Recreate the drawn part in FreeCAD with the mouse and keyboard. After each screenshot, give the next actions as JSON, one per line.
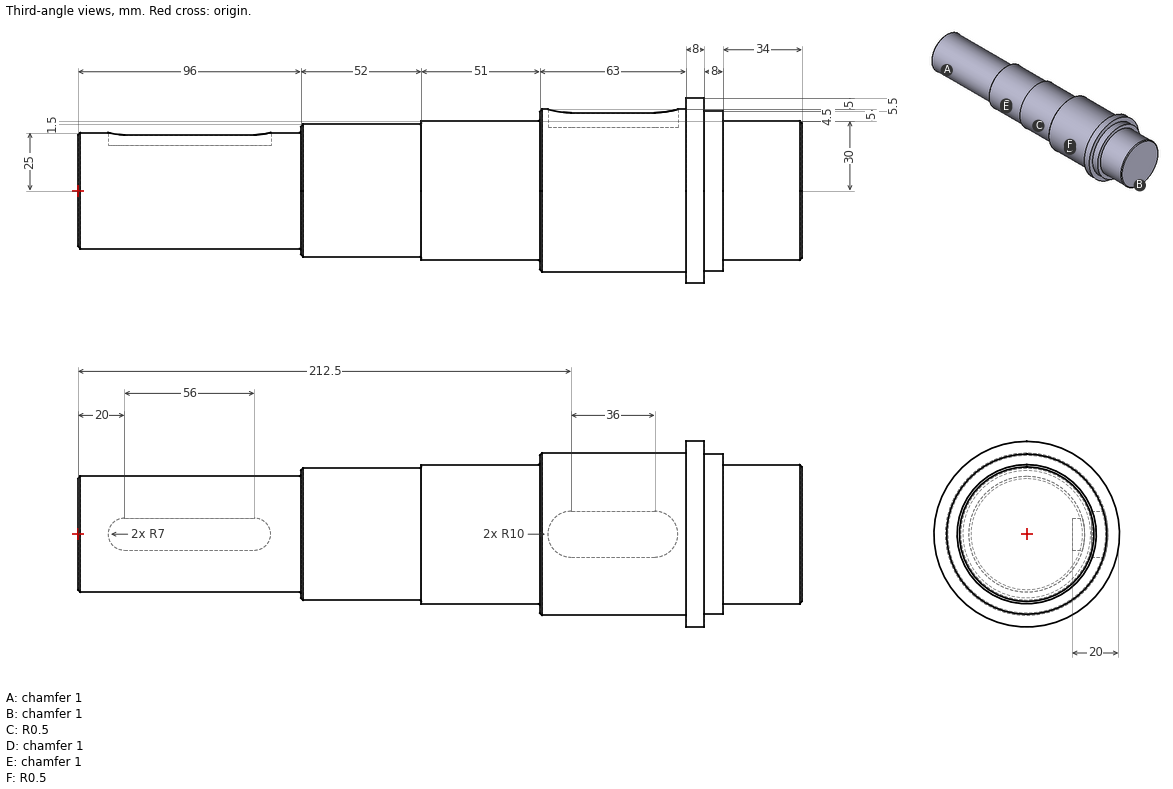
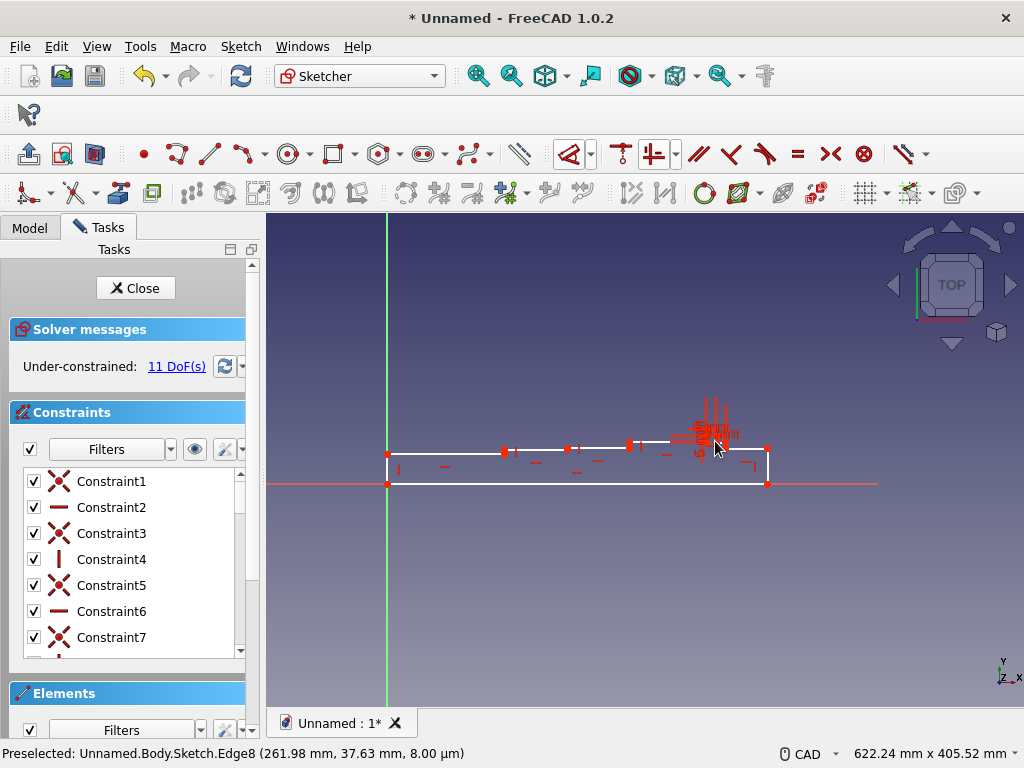
{"action": "scroll", "coordinate": [630, 444], "scroll_direction": "up", "scroll_amount": 11}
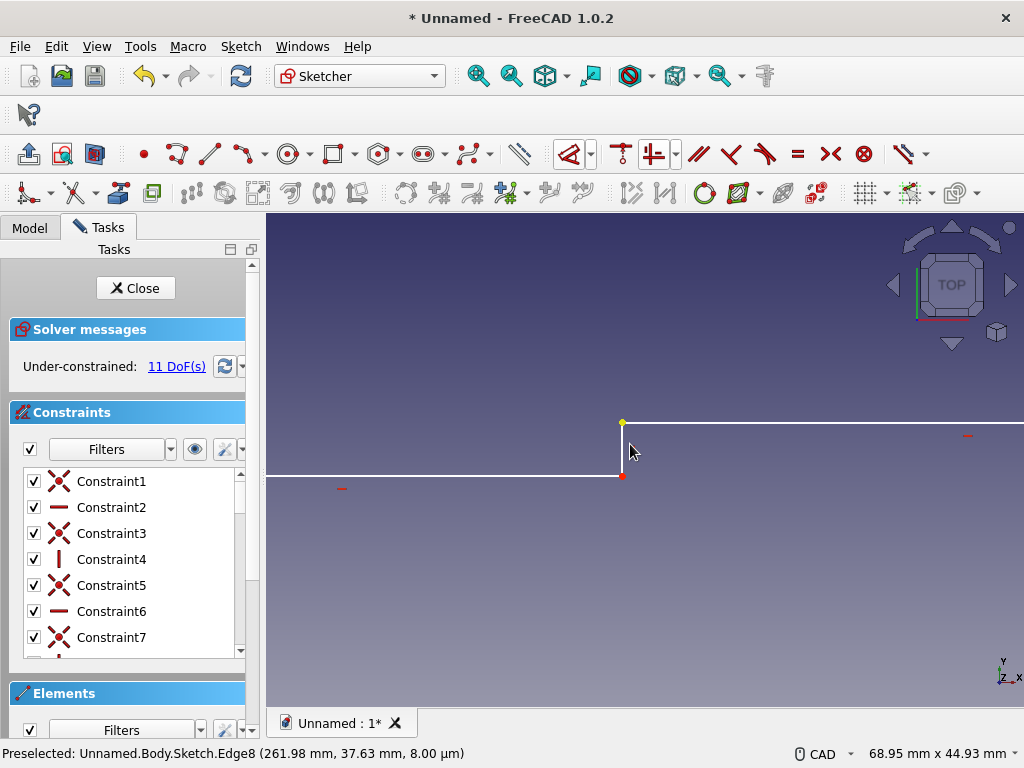
{"action": "left_click", "coordinate": [622, 439]}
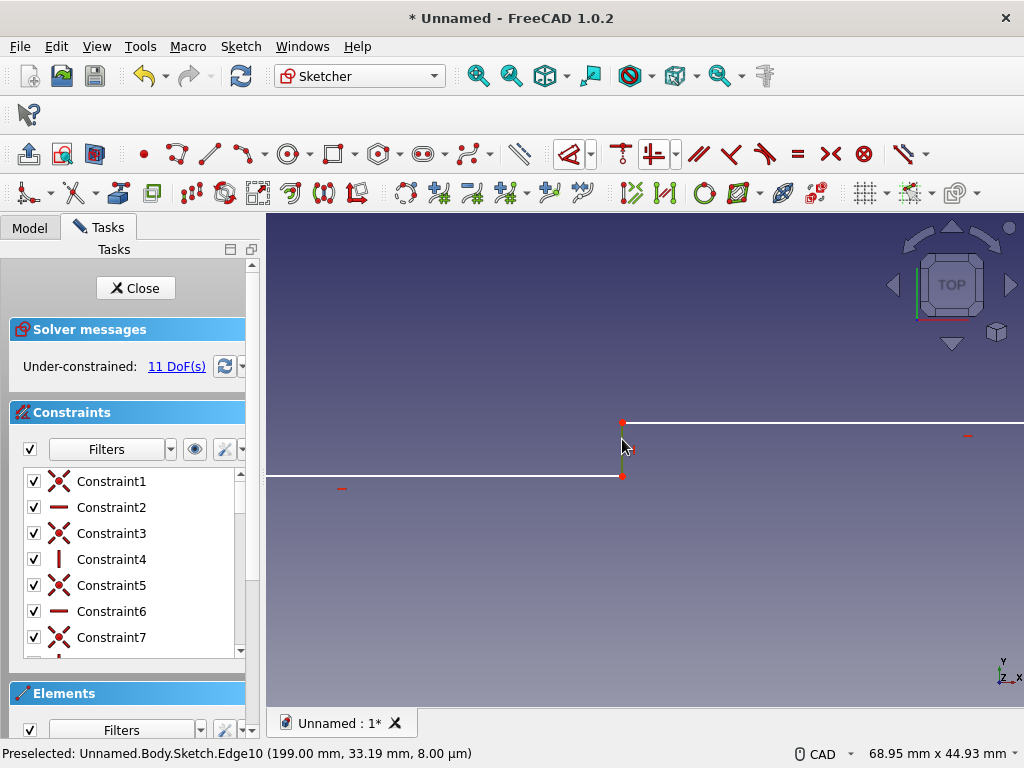
{"action": "key", "text": "i"}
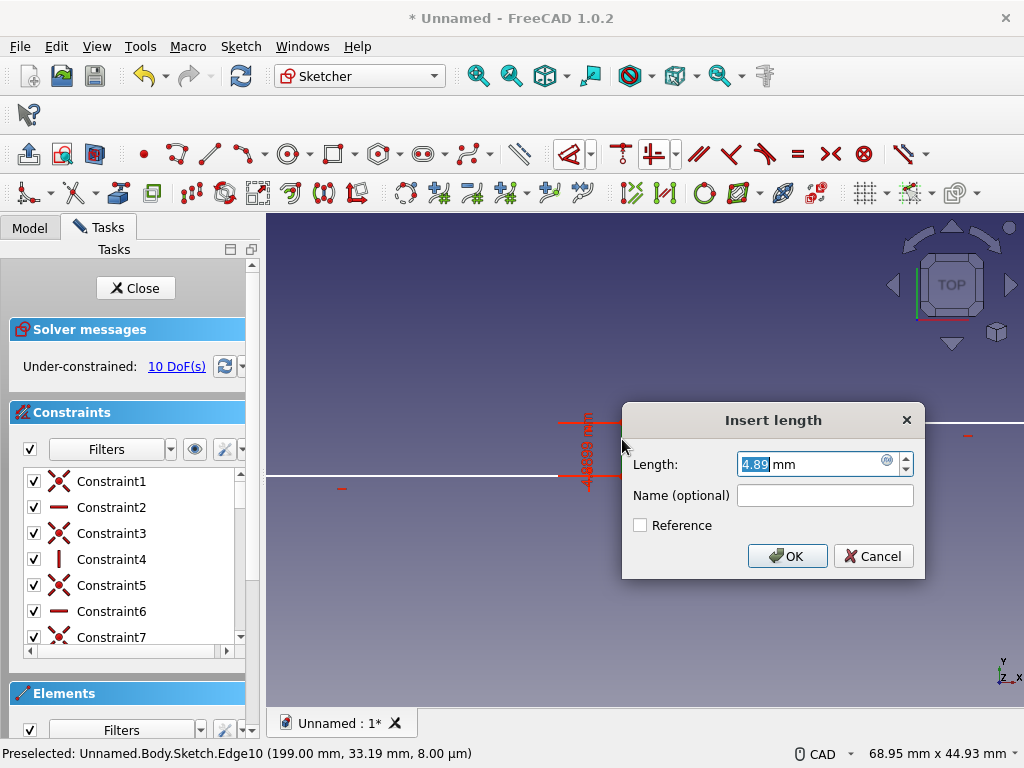
{"action": "type", "text": "5"}
{"action": "key", "text": "Return"}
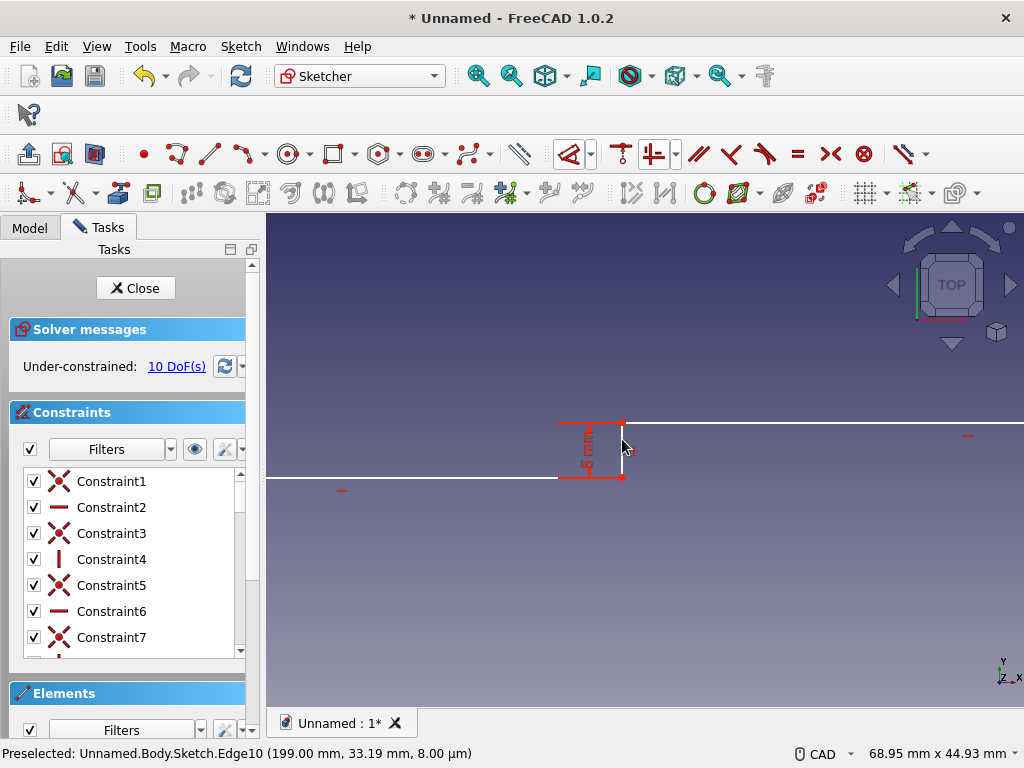
{"action": "scroll", "coordinate": [630, 444], "scroll_direction": "down", "scroll_amount": 11}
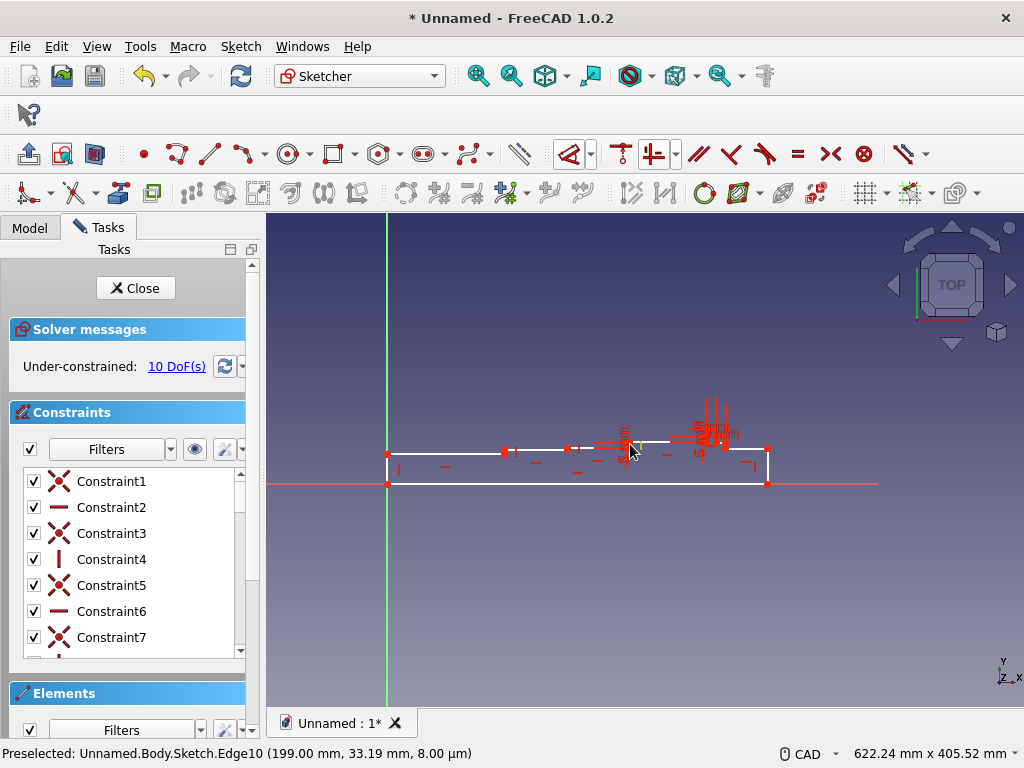
{"action": "scroll", "coordinate": [768, 474], "scroll_direction": "up", "scroll_amount": 2}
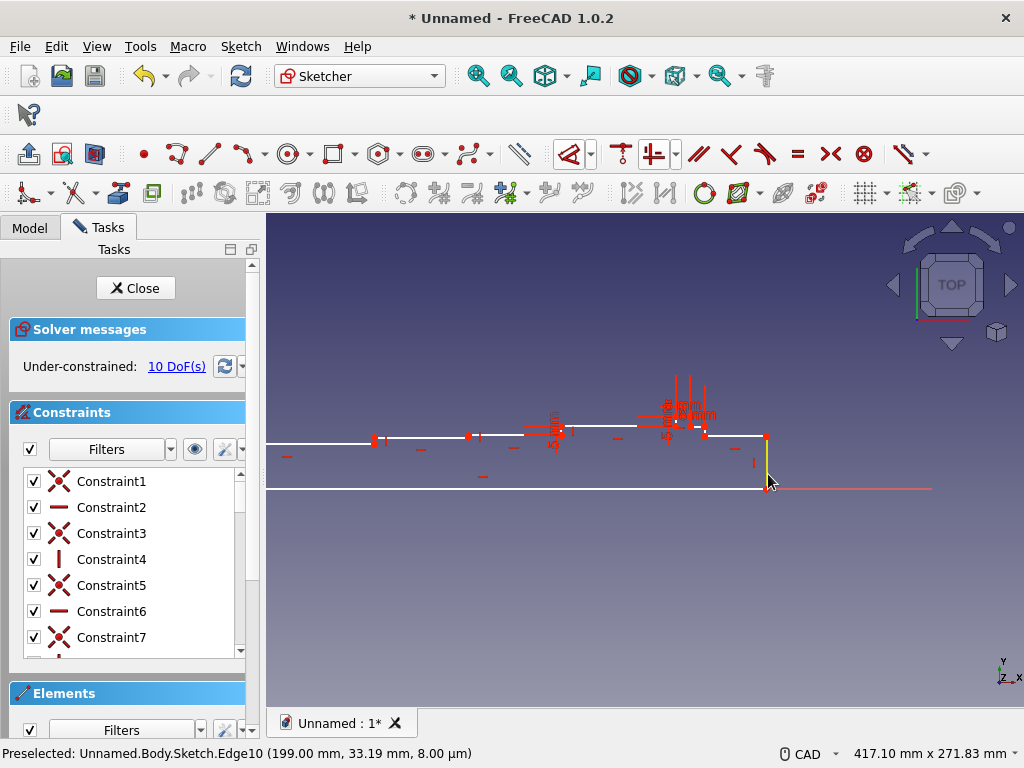
{"action": "left_click", "coordinate": [767, 473]}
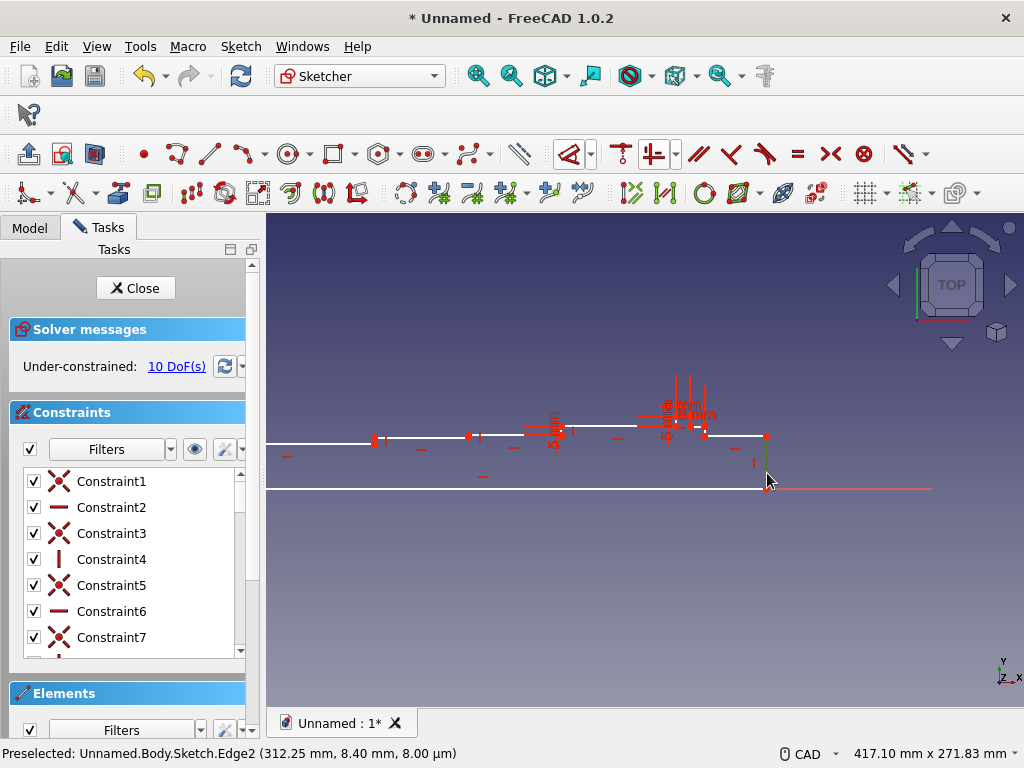
{"action": "key", "text": "i"}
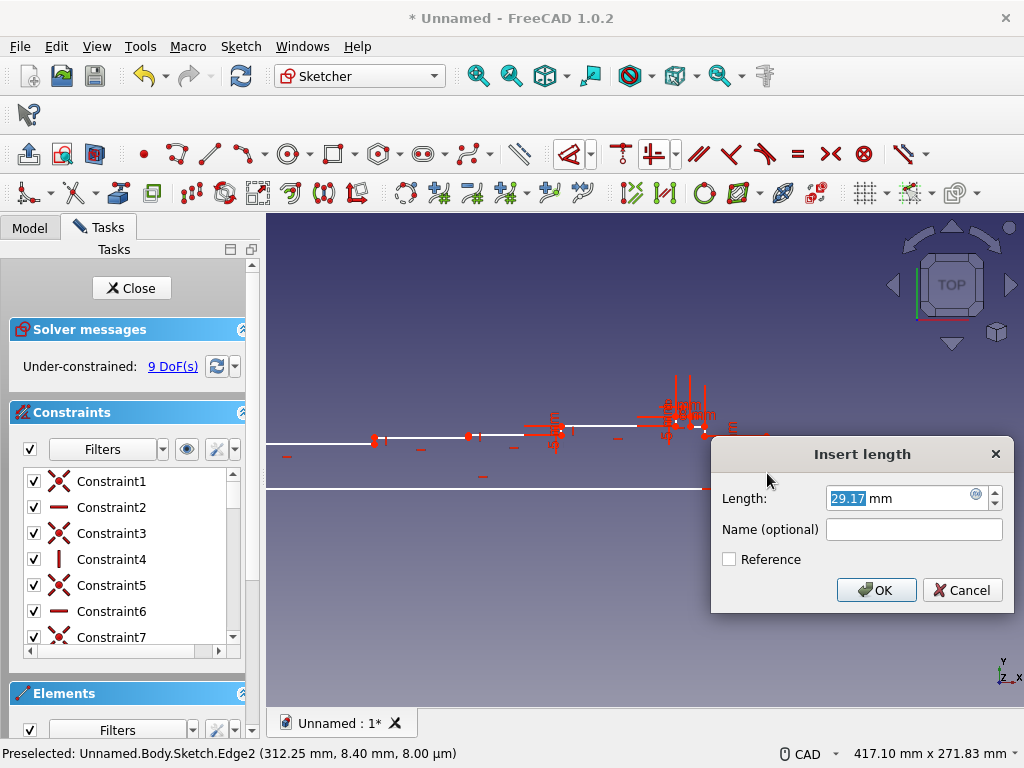
{"action": "type", "text": "30"}
{"action": "key", "text": "Return"}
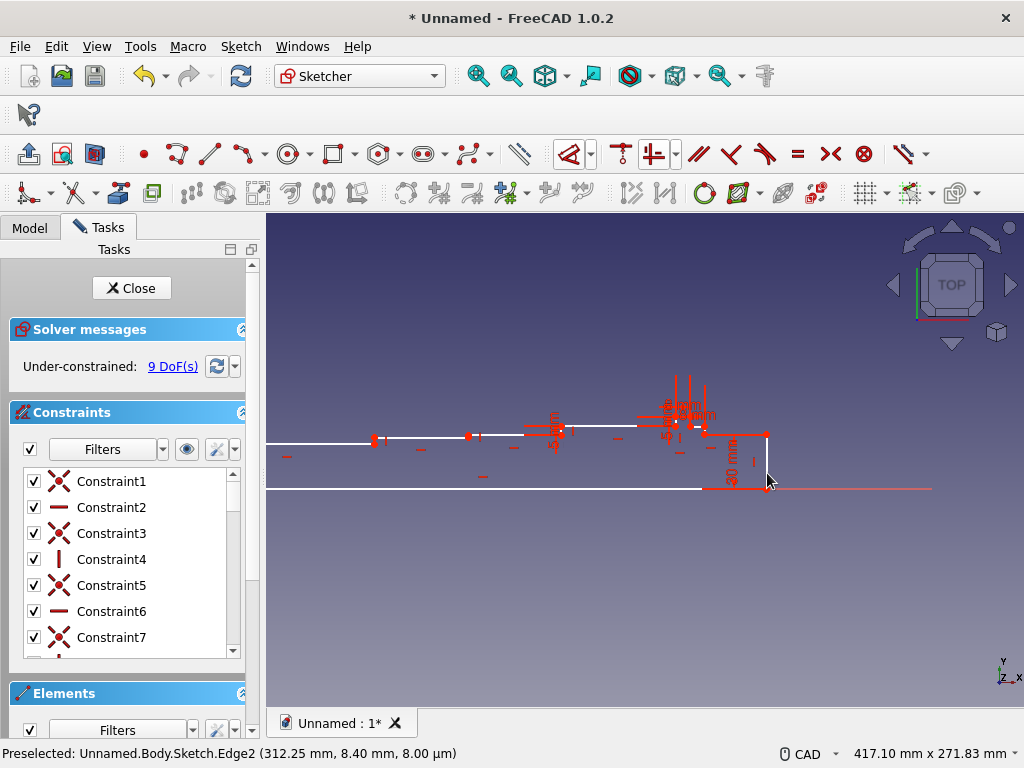
{"action": "left_click", "coordinate": [748, 435]}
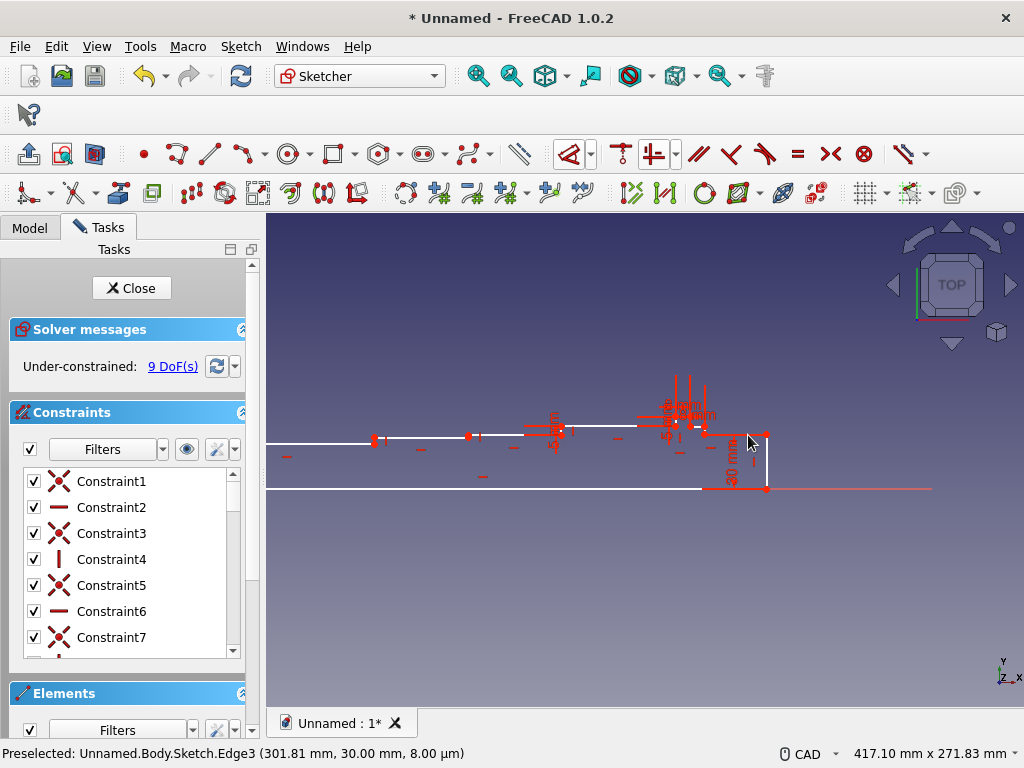
{"action": "left_click", "coordinate": [590, 154]}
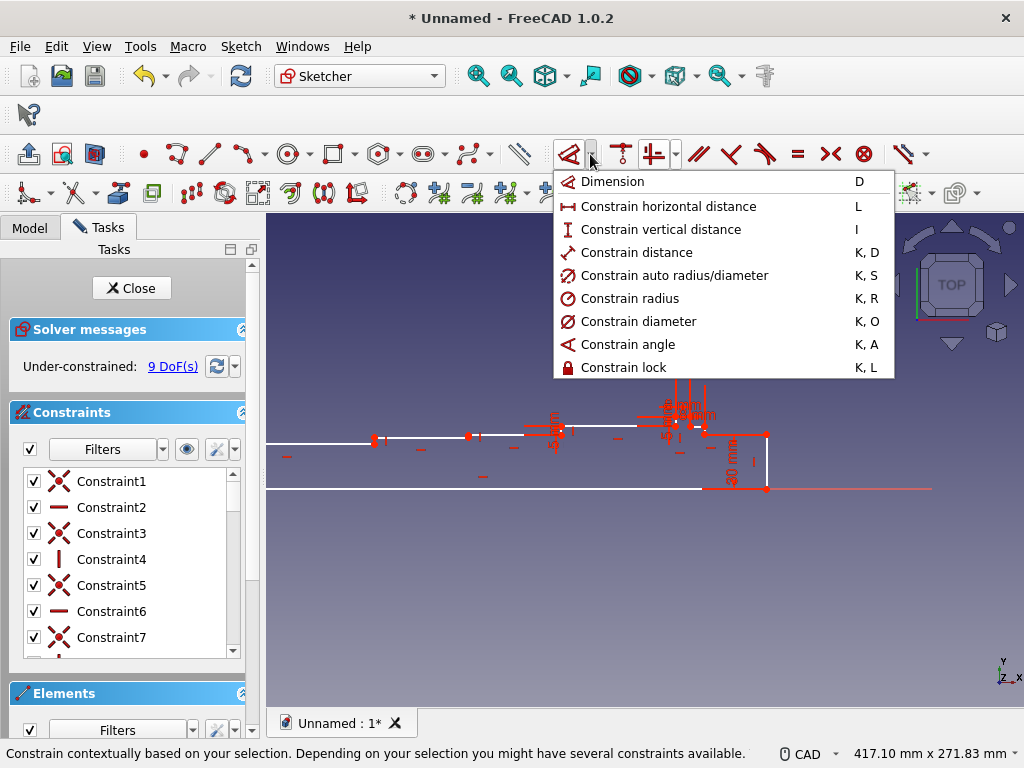
{"action": "left_click", "coordinate": [724, 206]}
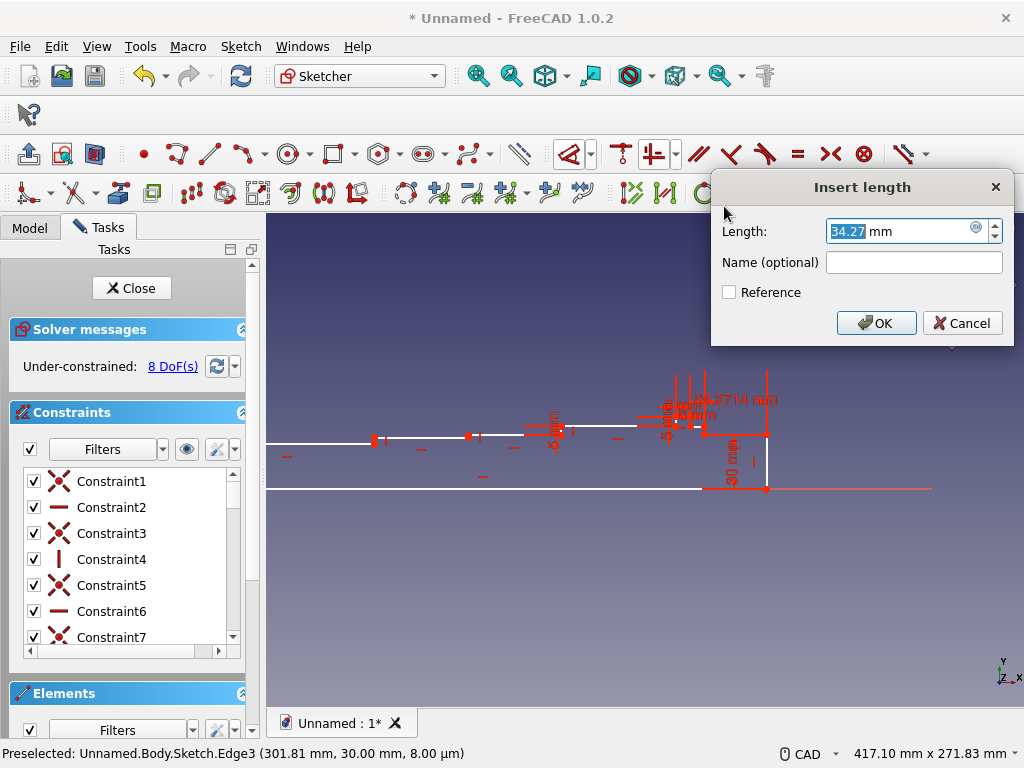
{"action": "type", "text": "34"}
{"action": "key", "text": "Return"}